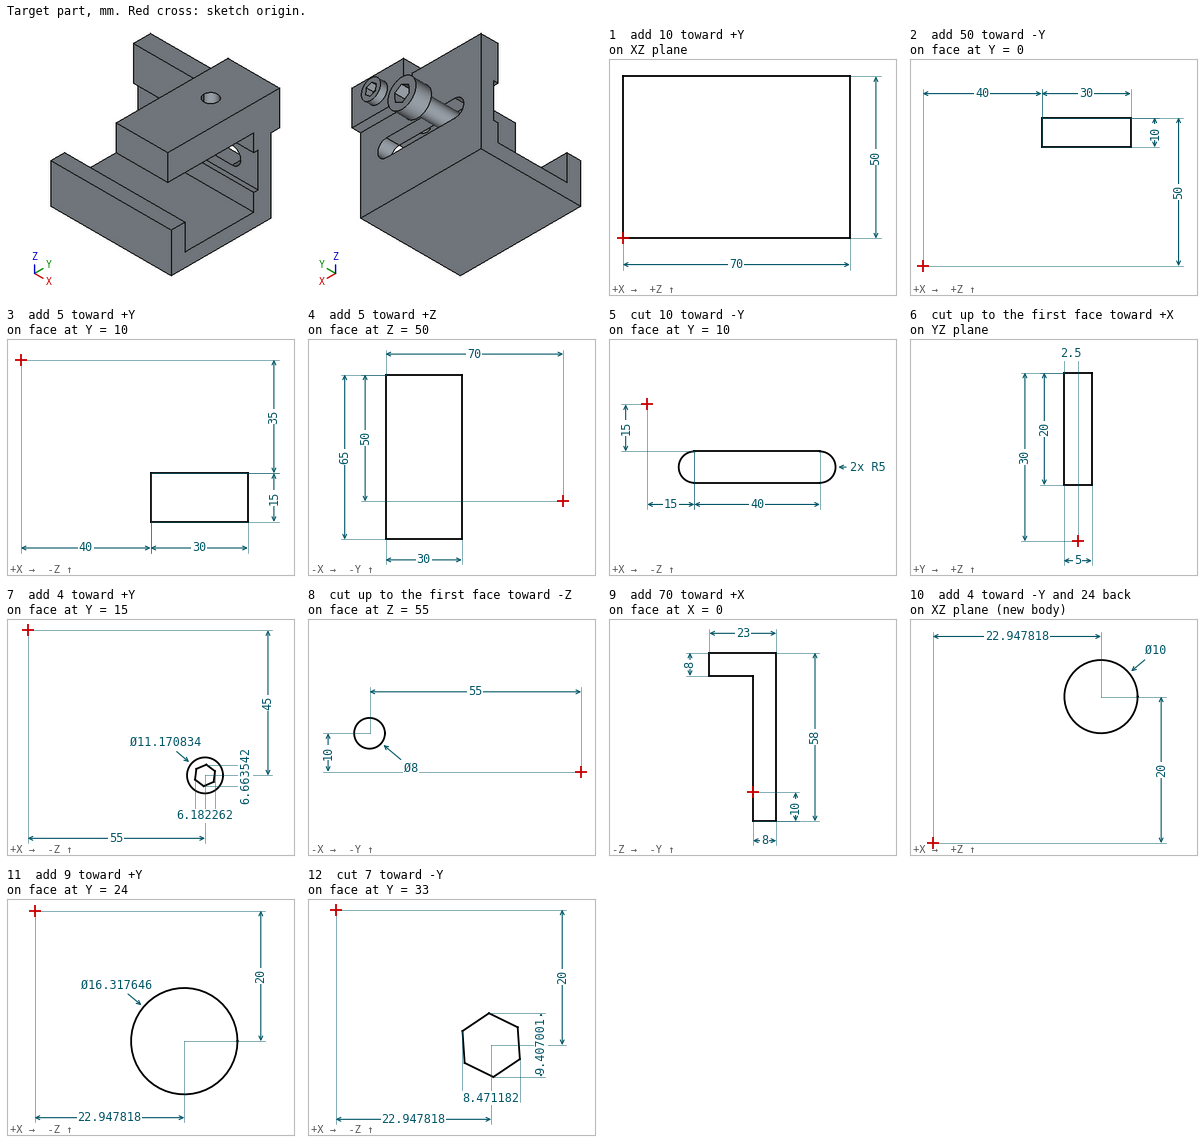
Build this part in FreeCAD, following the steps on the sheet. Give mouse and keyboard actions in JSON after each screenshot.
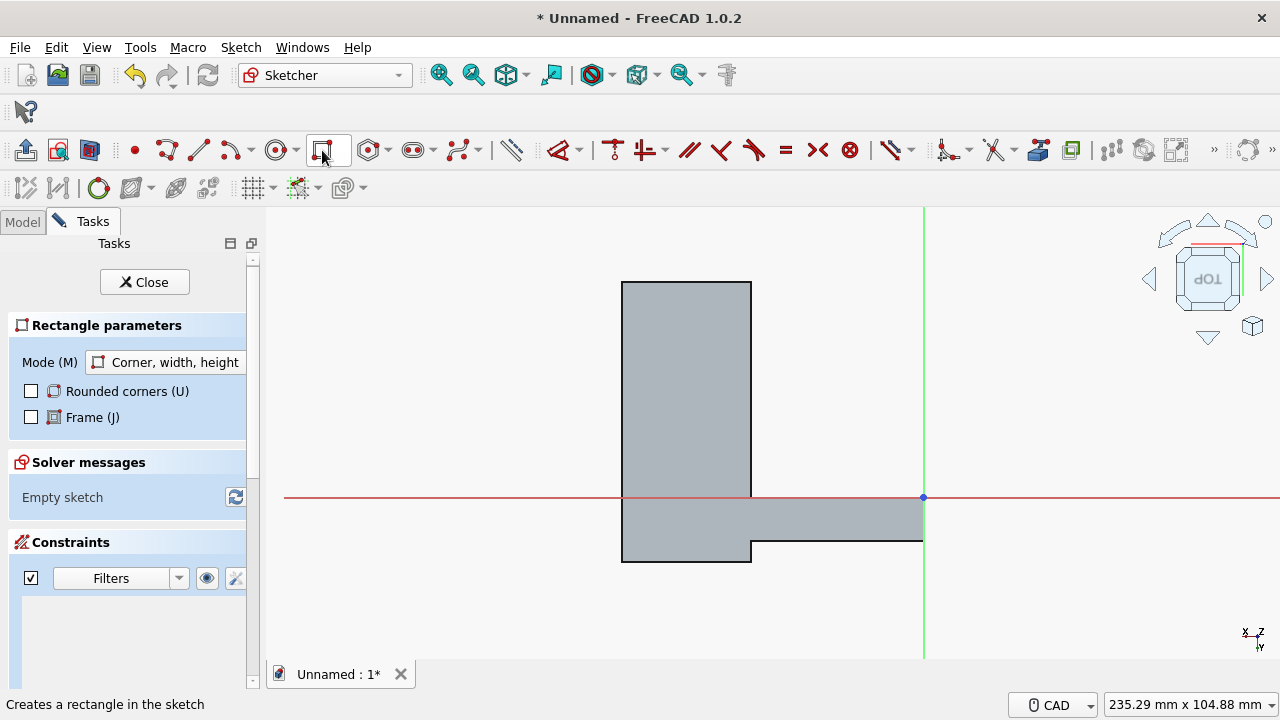
{"action": "left_click", "coordinate": [622, 282]}
{"action": "left_click", "coordinate": [751, 562]}
{"action": "key", "text": "Escape"}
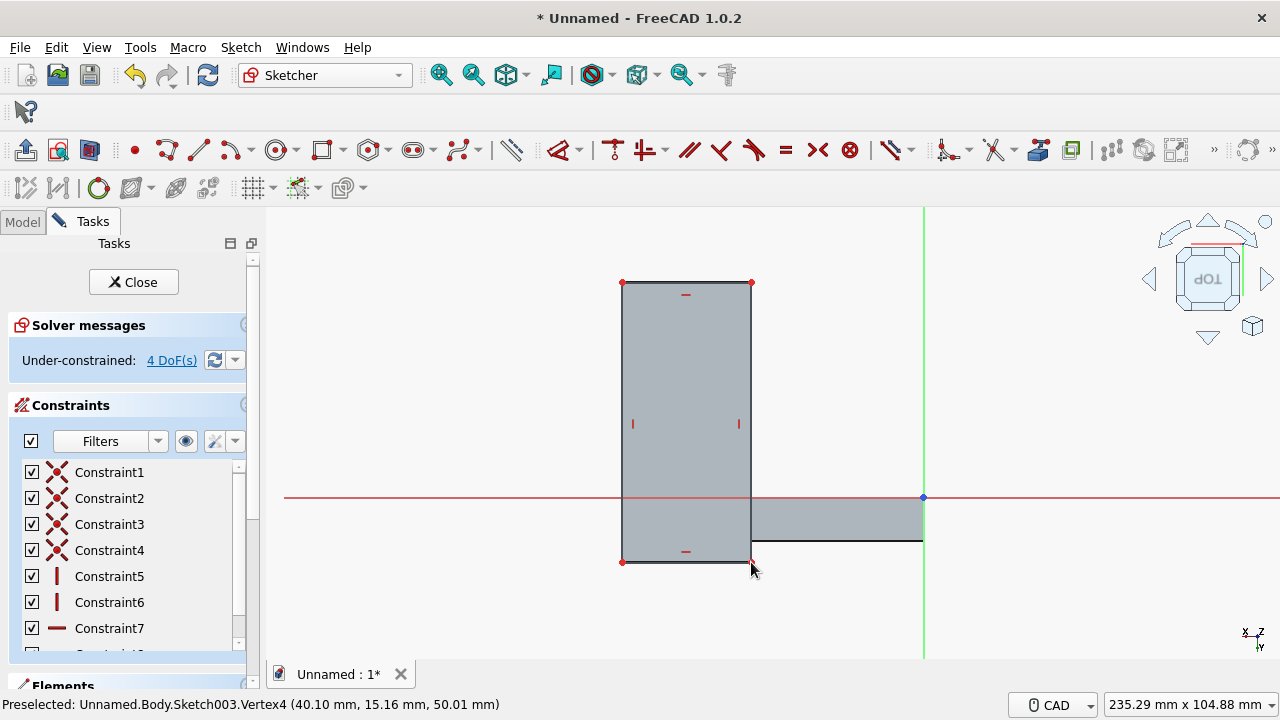
{"action": "left_click", "coordinate": [558, 150]}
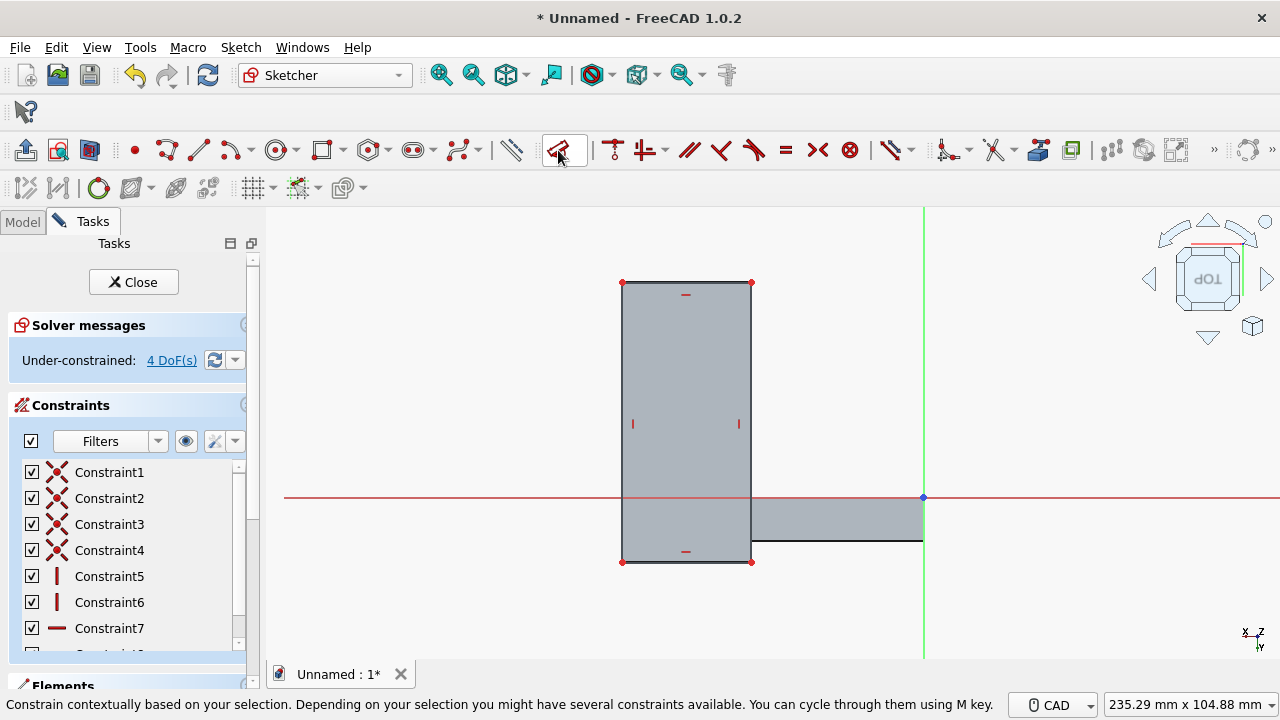
{"action": "left_click", "coordinate": [622, 367]}
{"action": "left_click", "coordinate": [588, 423]}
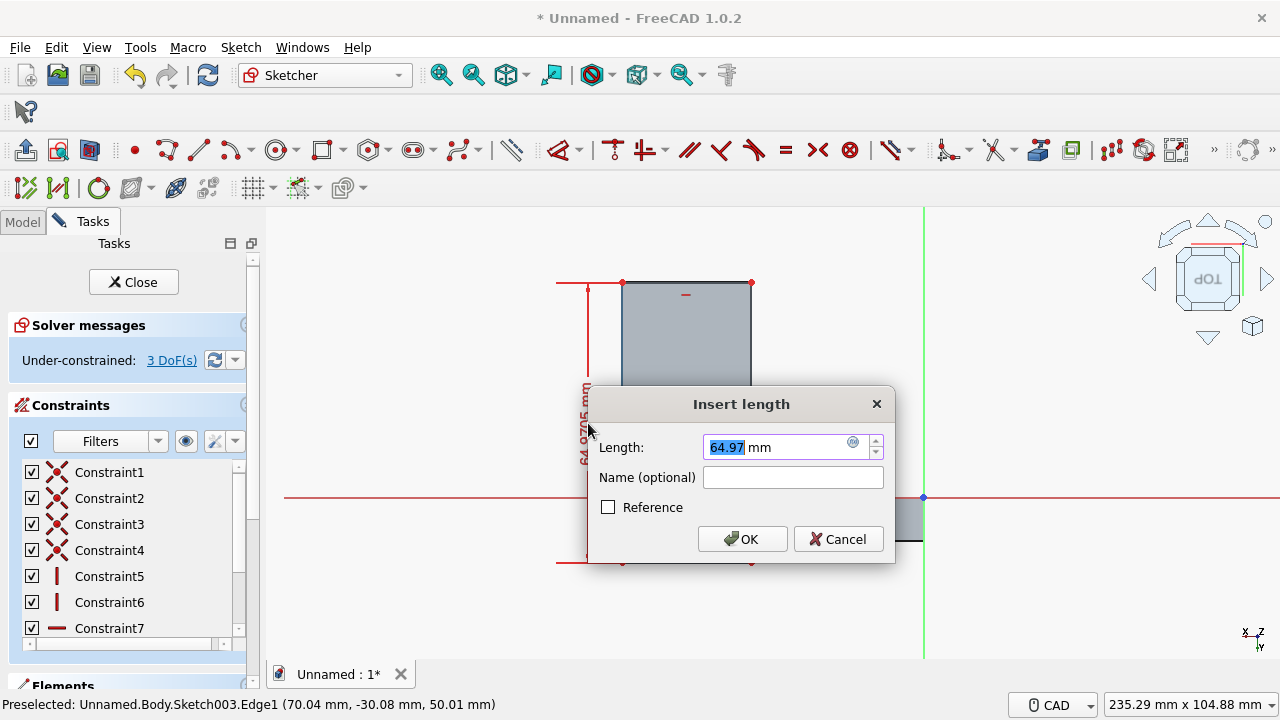
{"action": "type", "text": "65"}
{"action": "key", "text": "Return"}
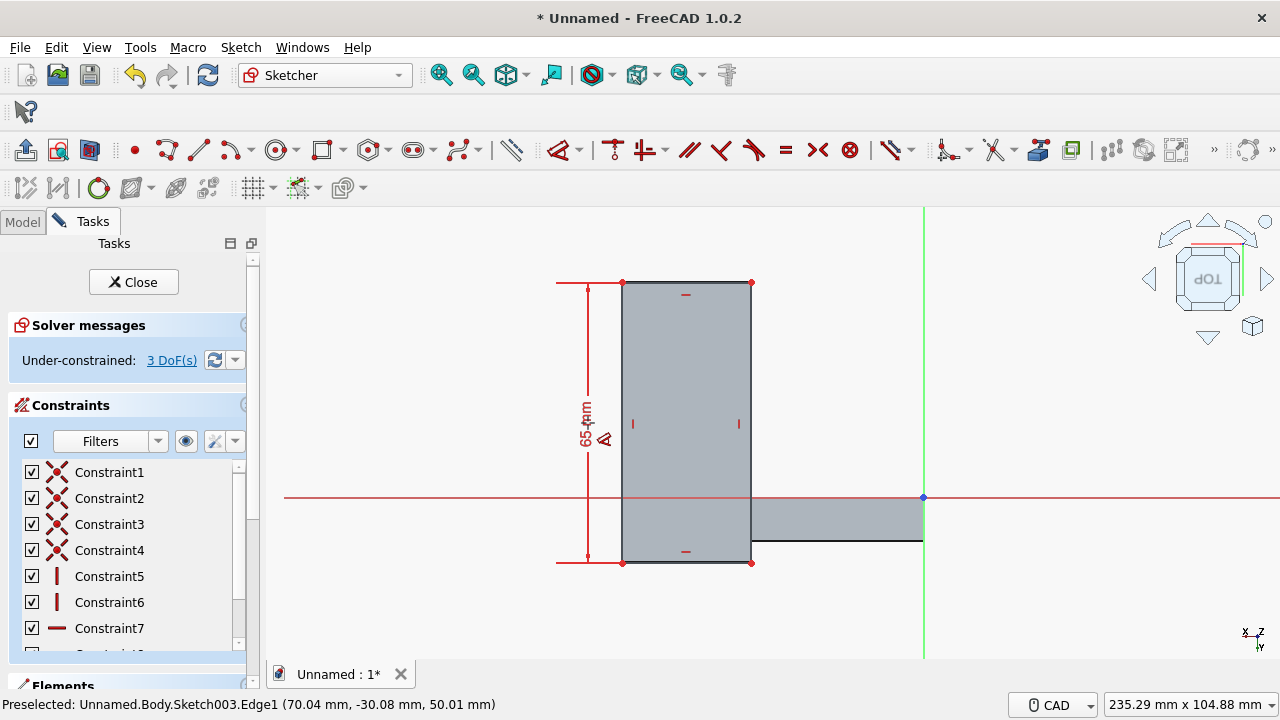
{"action": "left_click", "coordinate": [661, 563]}
{"action": "left_click", "coordinate": [686, 597]}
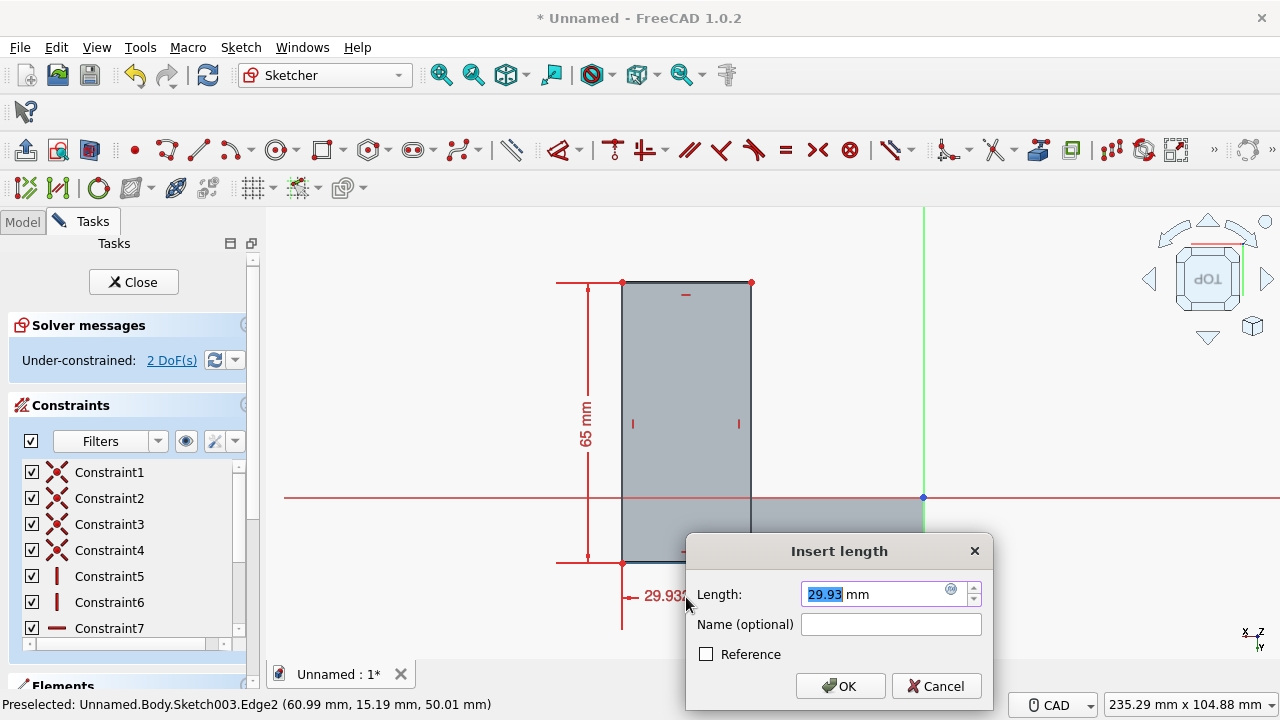
{"action": "type", "text": "30"}
{"action": "key", "text": "Return"}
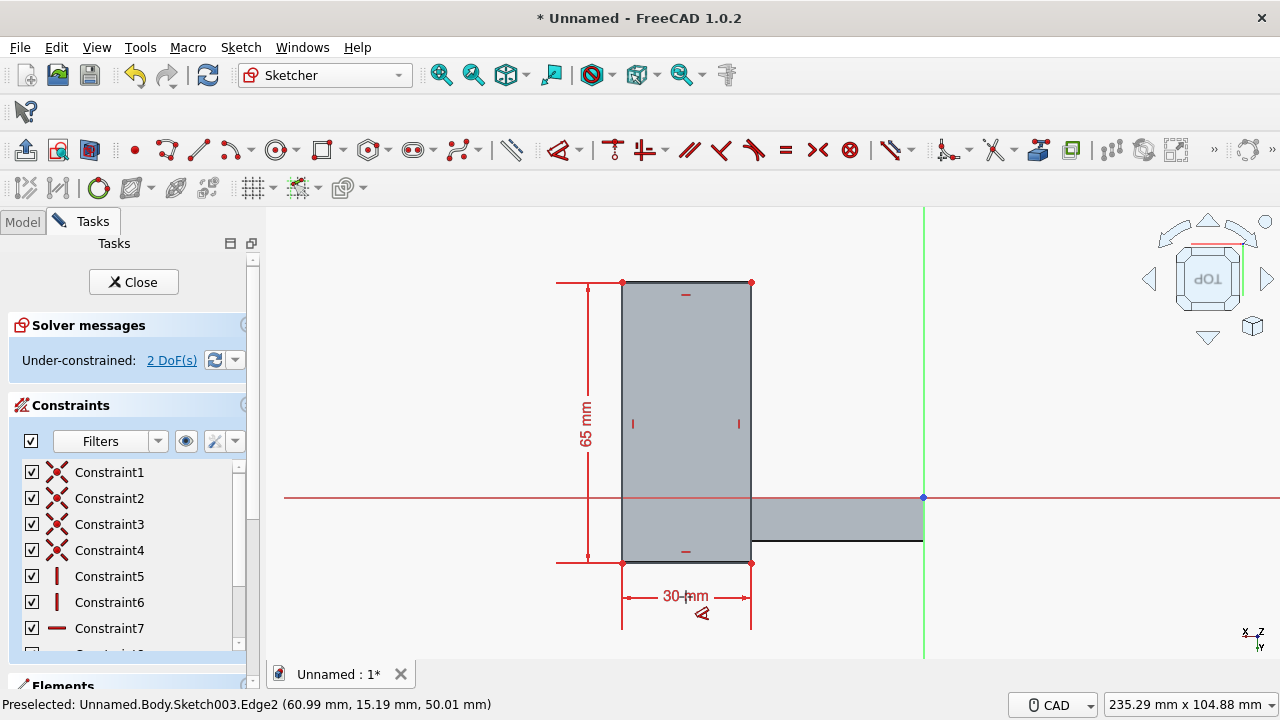
{"action": "left_click", "coordinate": [622, 283]}
{"action": "left_click", "coordinate": [773, 249]}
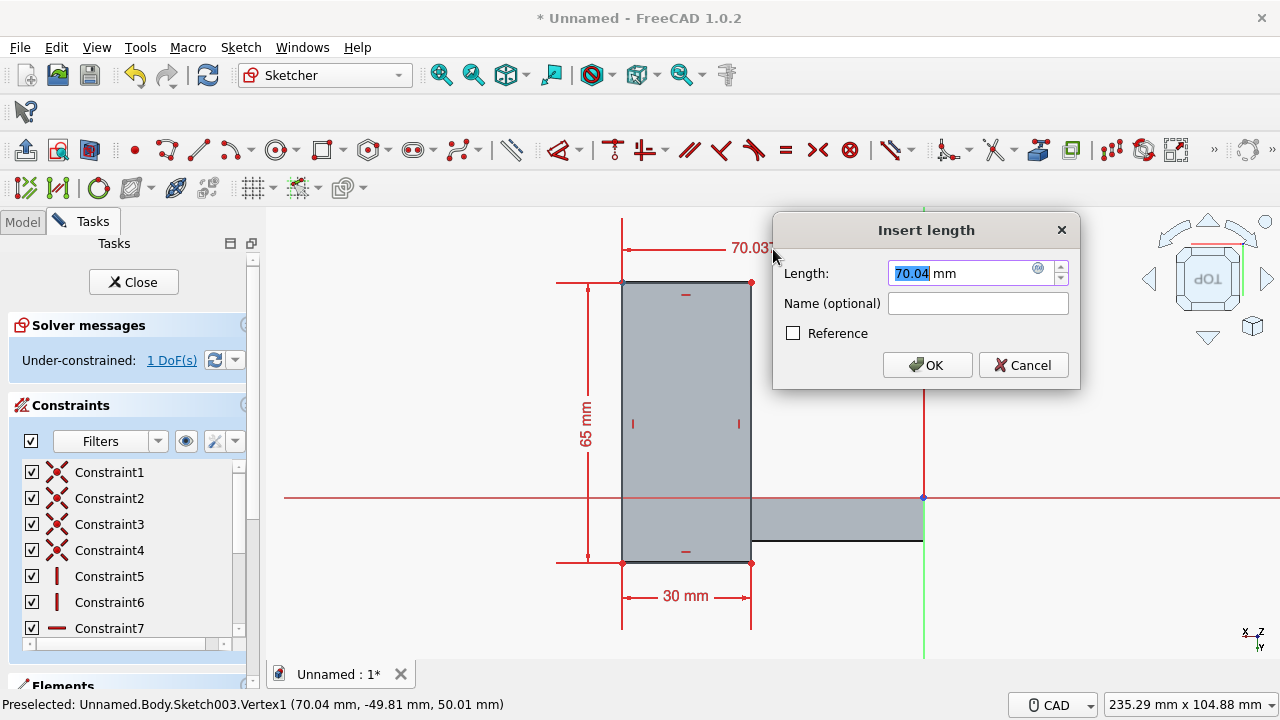
{"action": "type", "text": "70"}
{"action": "key", "text": "Return"}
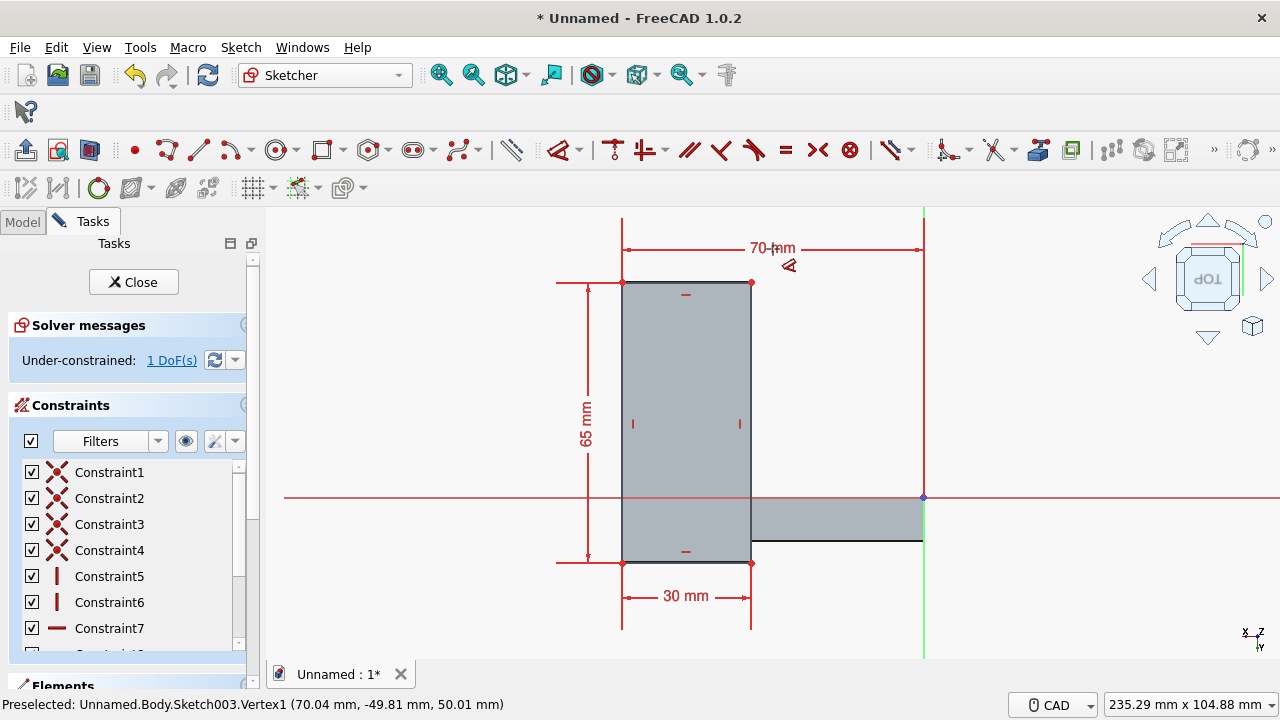
{"action": "left_click", "coordinate": [622, 283]}
{"action": "left_click", "coordinate": [958, 390]}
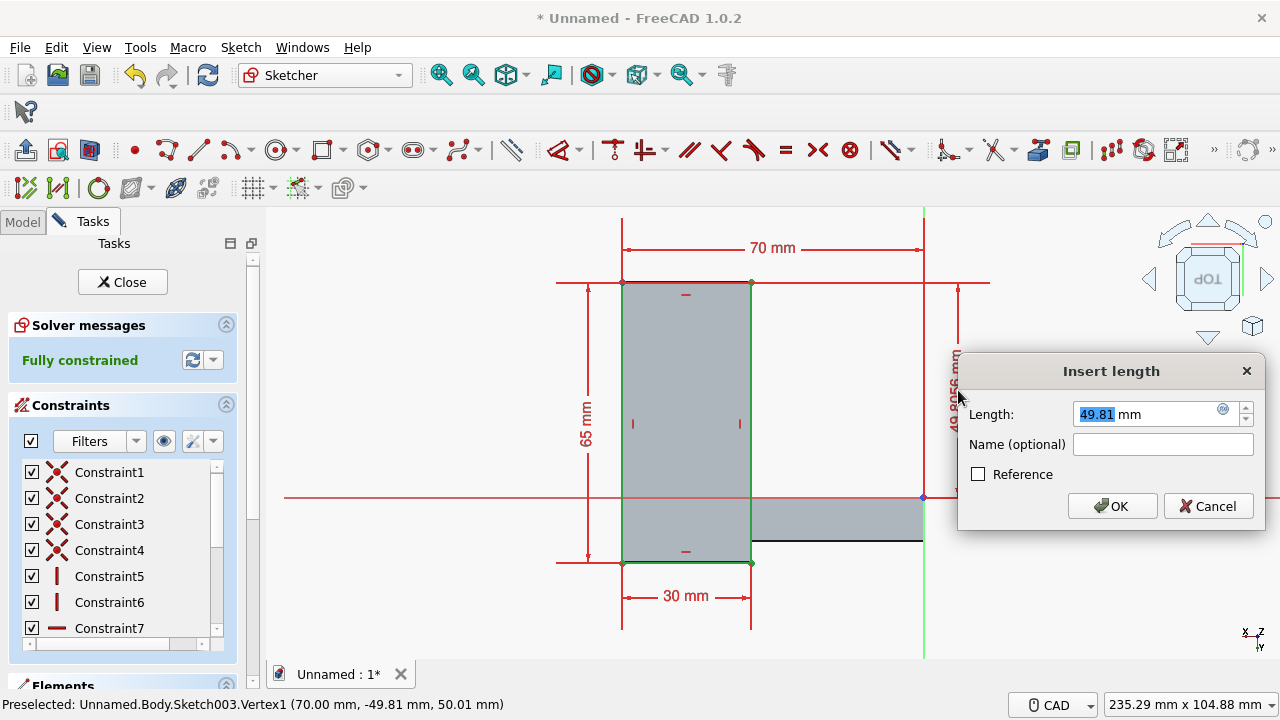
{"action": "type", "text": "50"}
{"action": "key", "text": "Return"}
{"action": "key", "text": "Escape"}